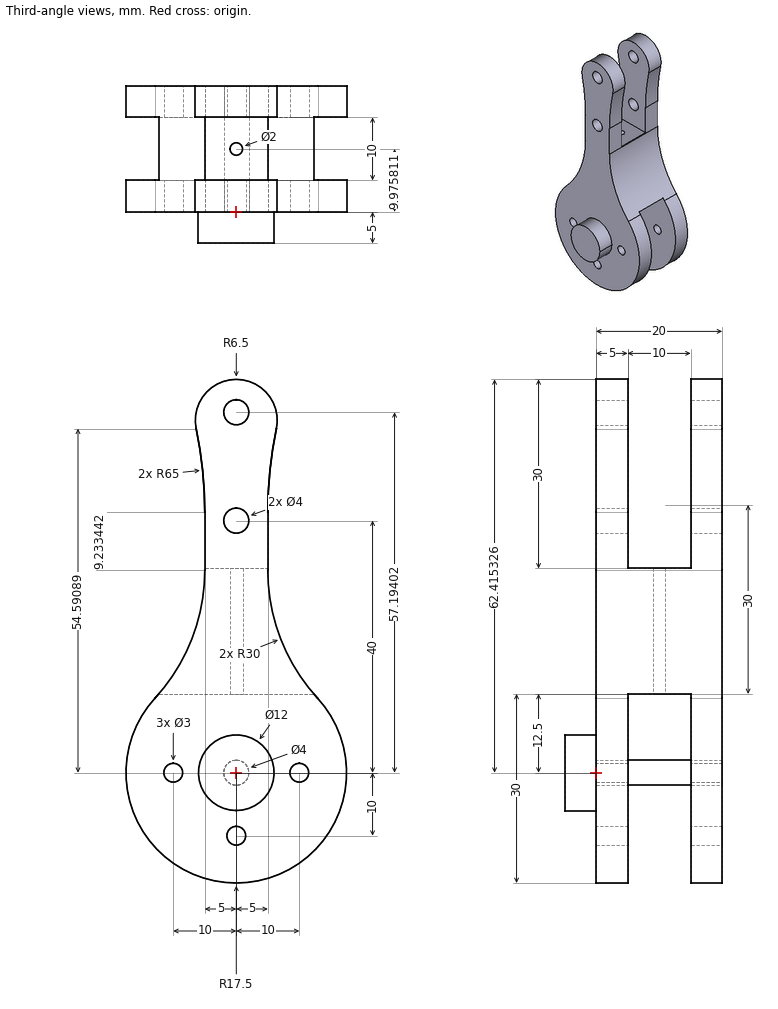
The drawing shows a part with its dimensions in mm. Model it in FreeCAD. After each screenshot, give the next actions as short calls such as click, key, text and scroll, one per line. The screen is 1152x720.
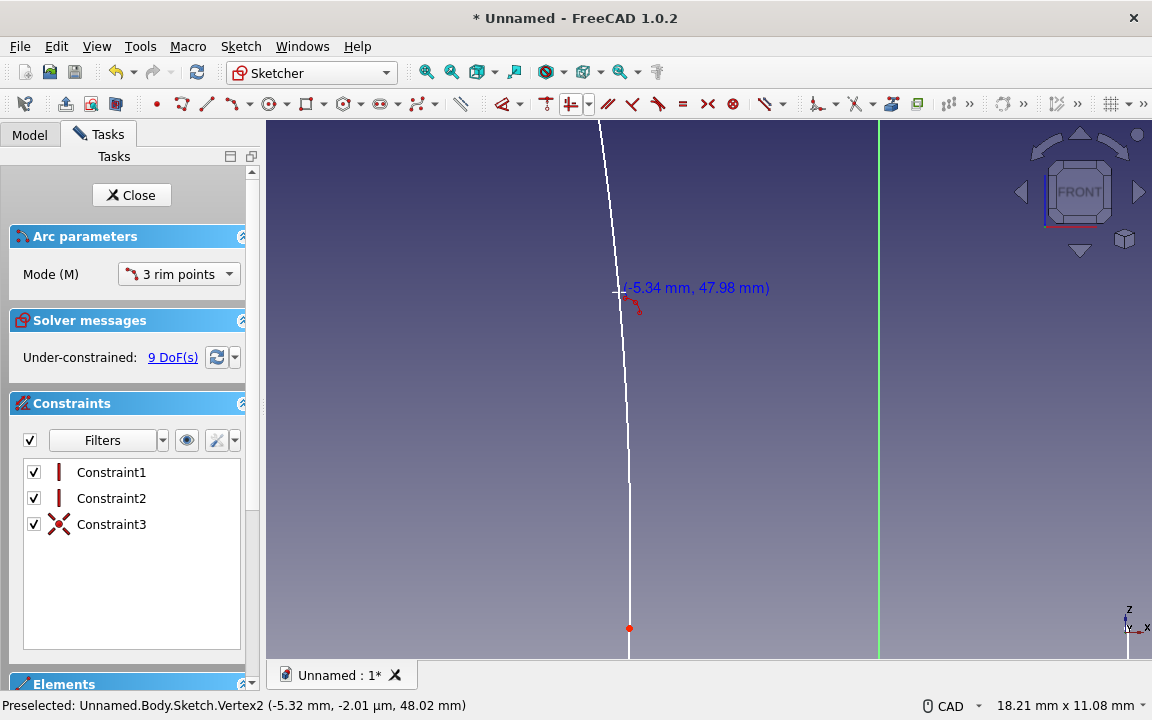
scroll(617, 275, down, 12)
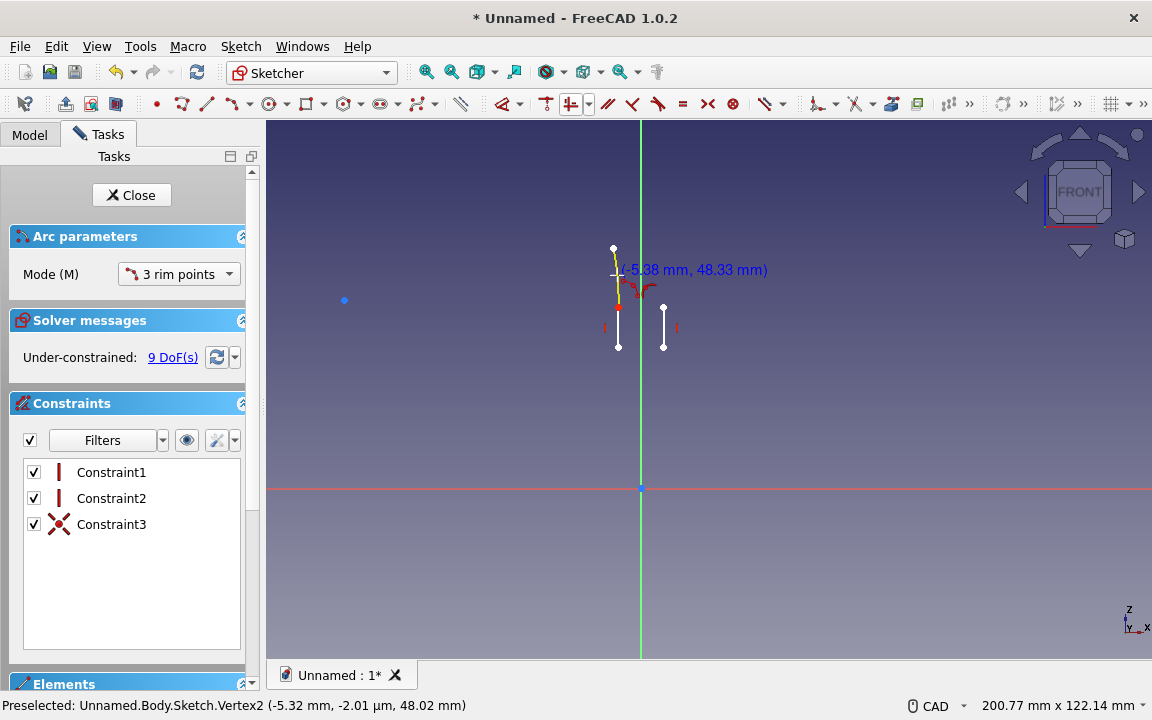
click(614, 249)
click(669, 248)
click(660, 220)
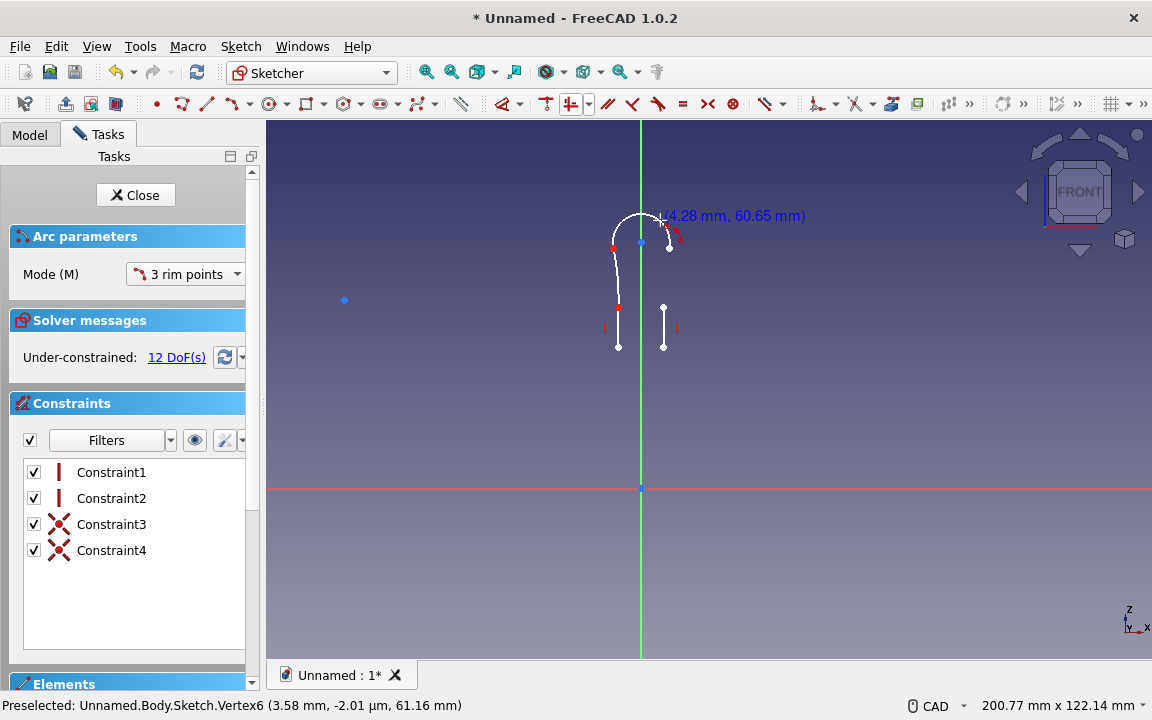
click(669, 249)
click(664, 307)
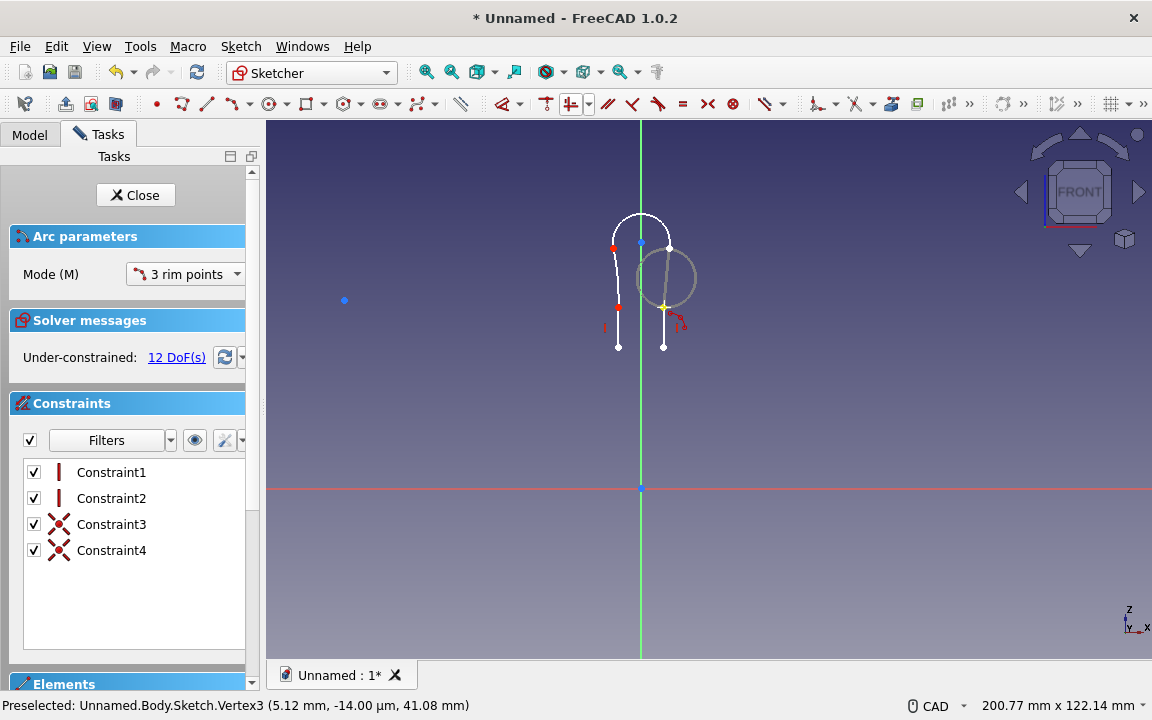
scroll(665, 277, up, 12)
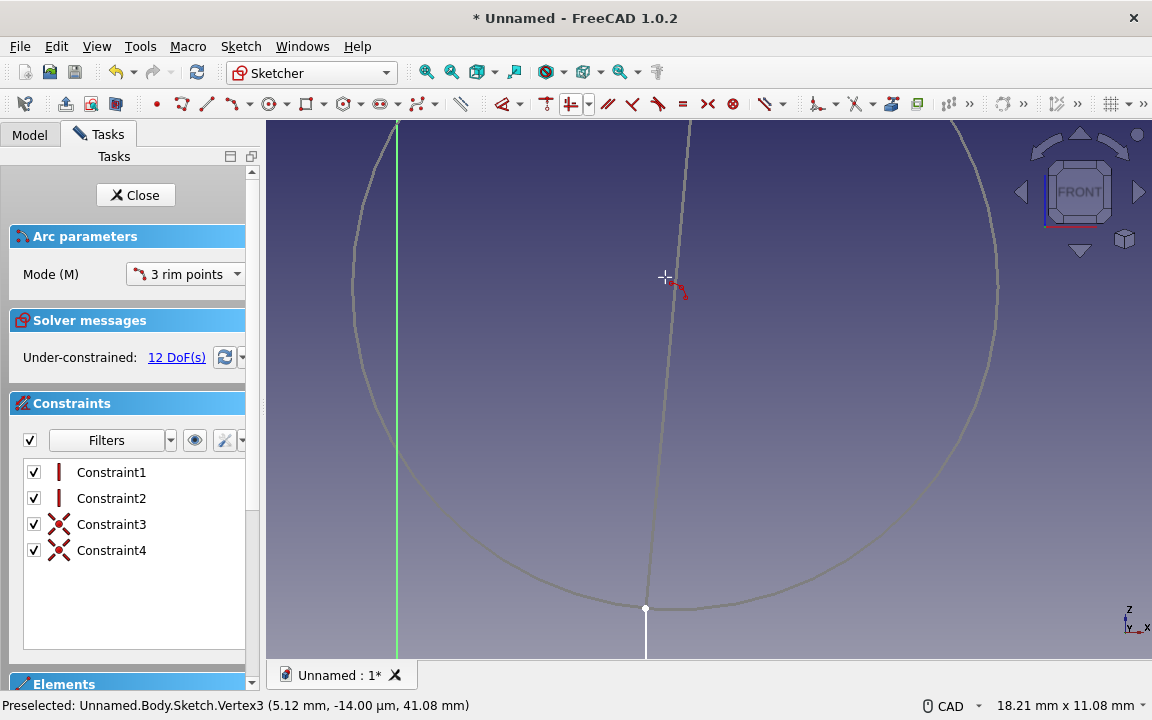
click(657, 272)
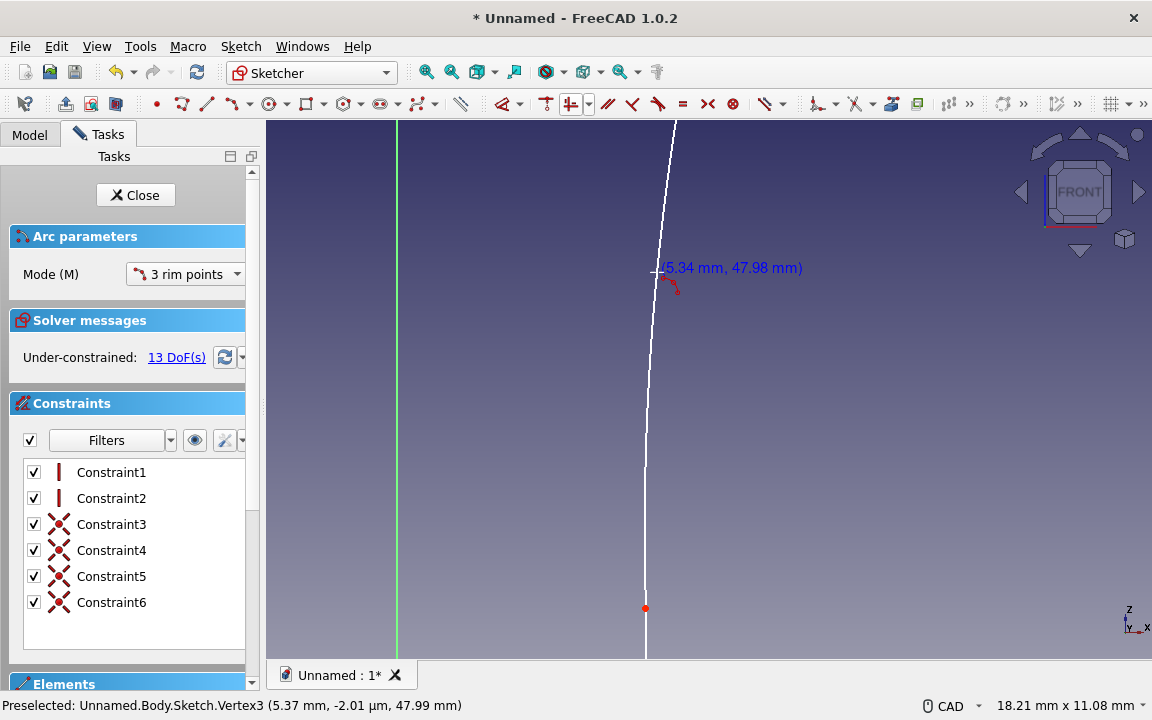
scroll(665, 277, down, 12)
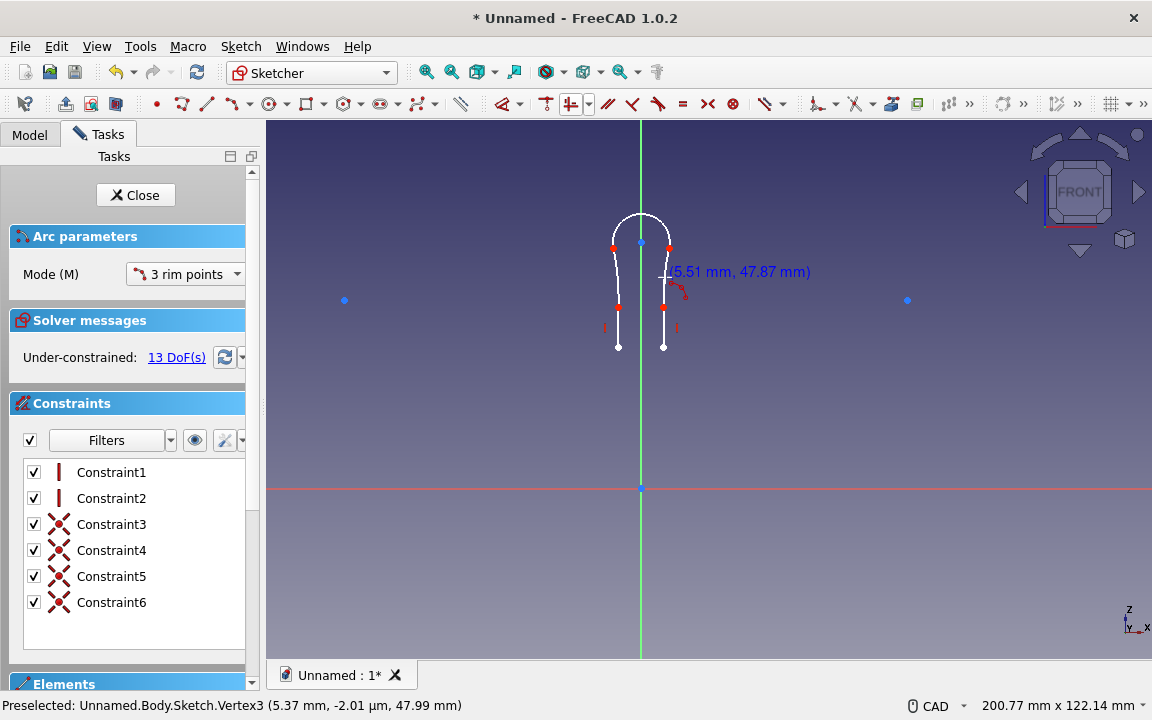
click(664, 348)
click(698, 436)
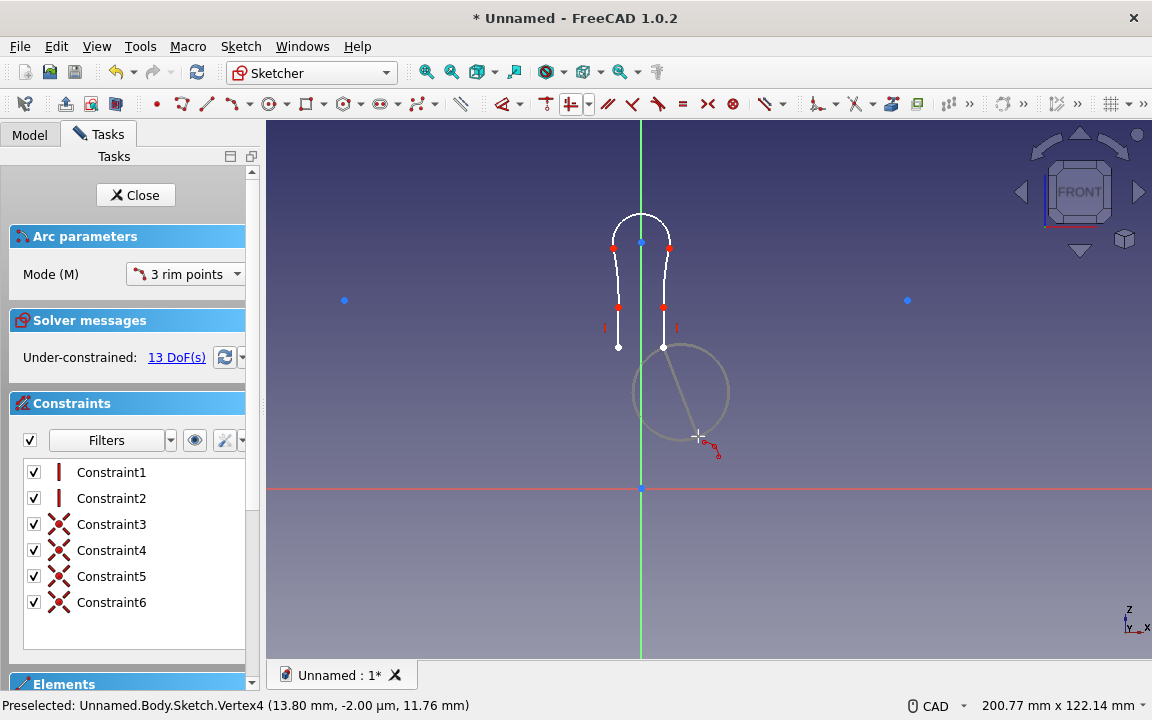
scroll(672, 395, up, 3)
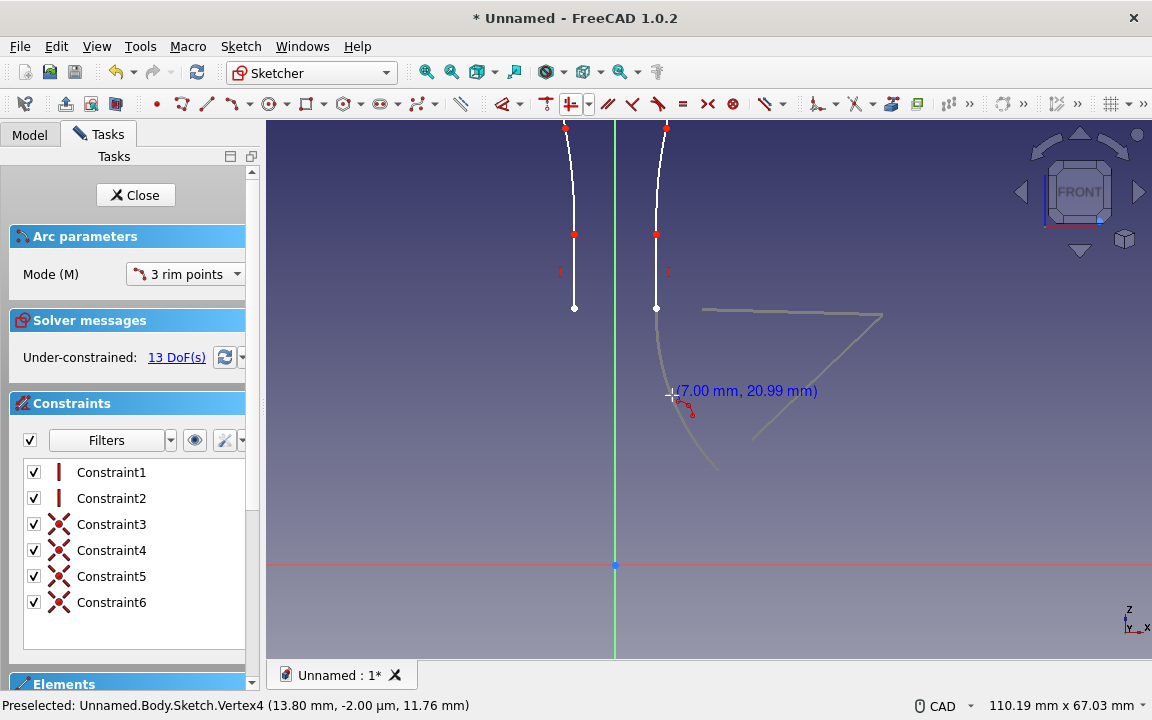
click(672, 394)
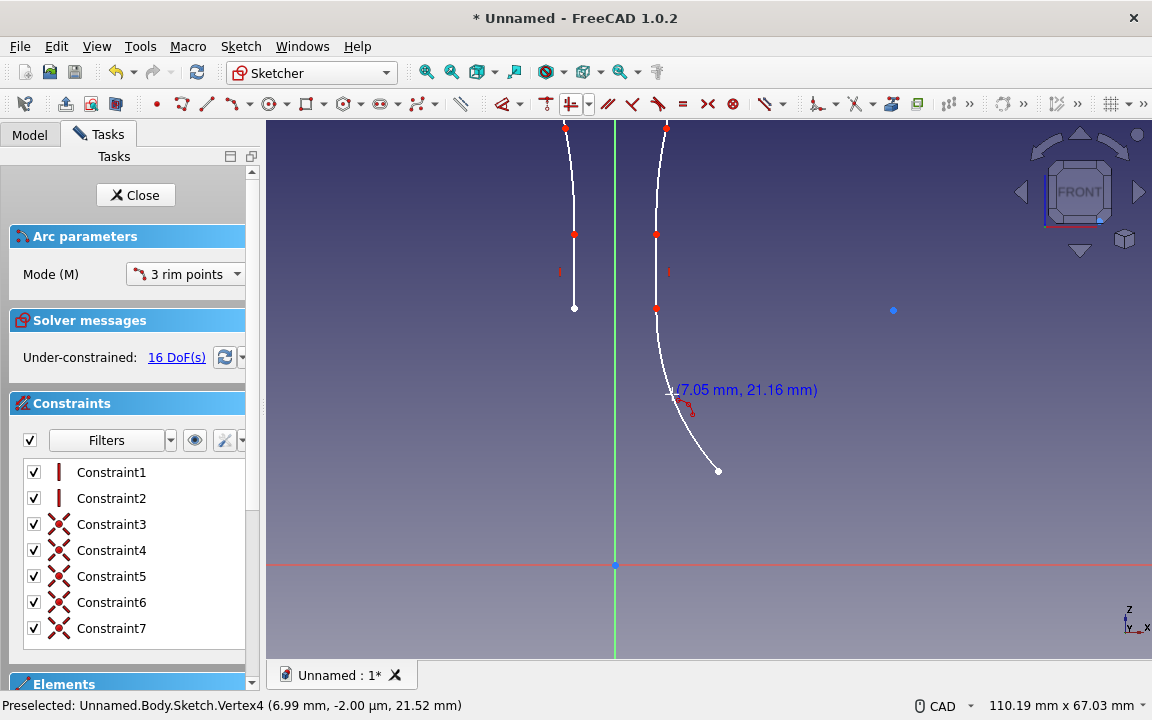
click(719, 471)
click(512, 470)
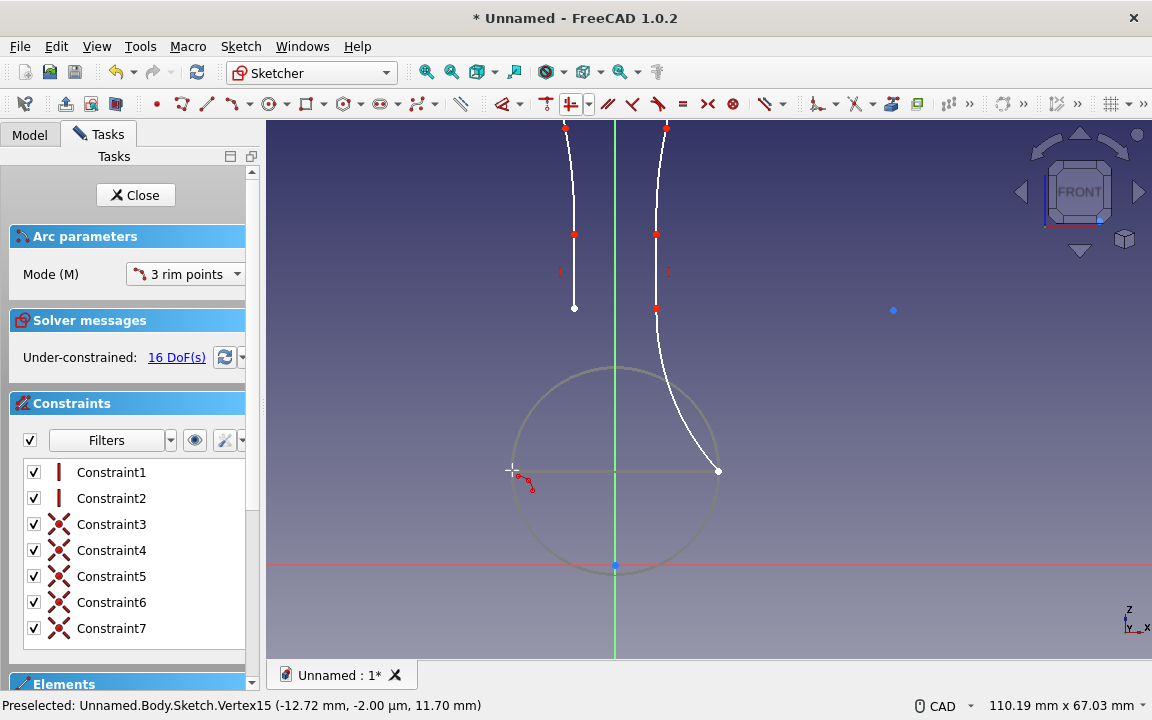
scroll(671, 395, down, 3)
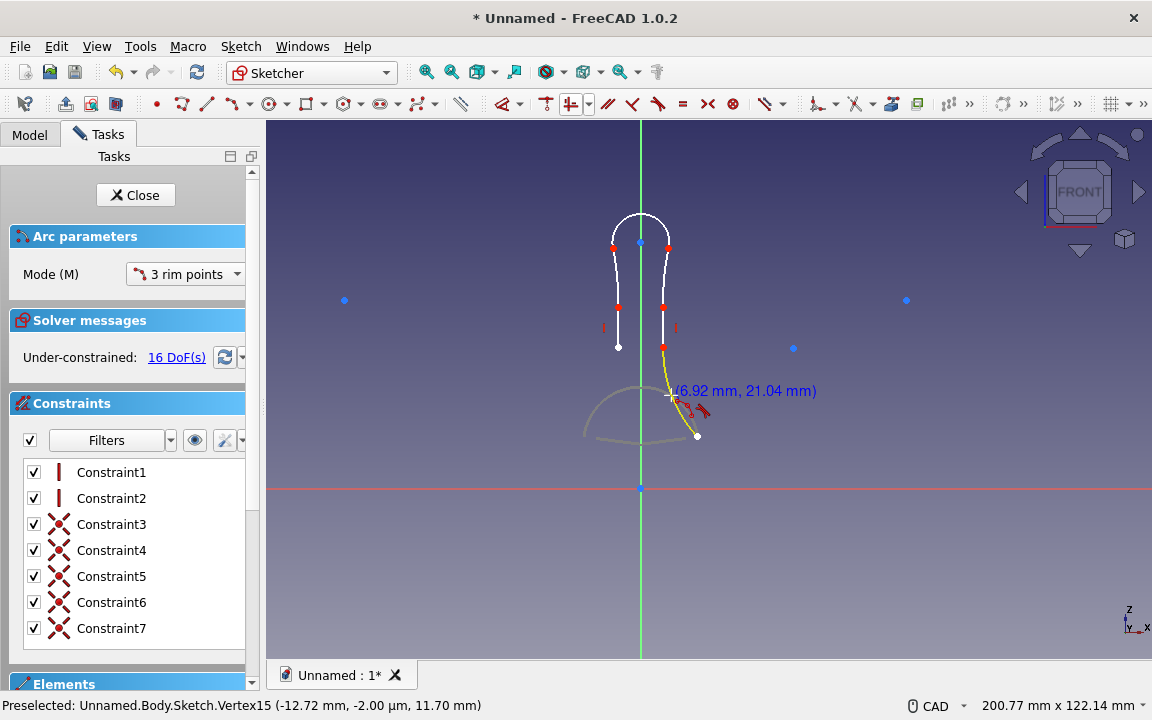
click(606, 558)